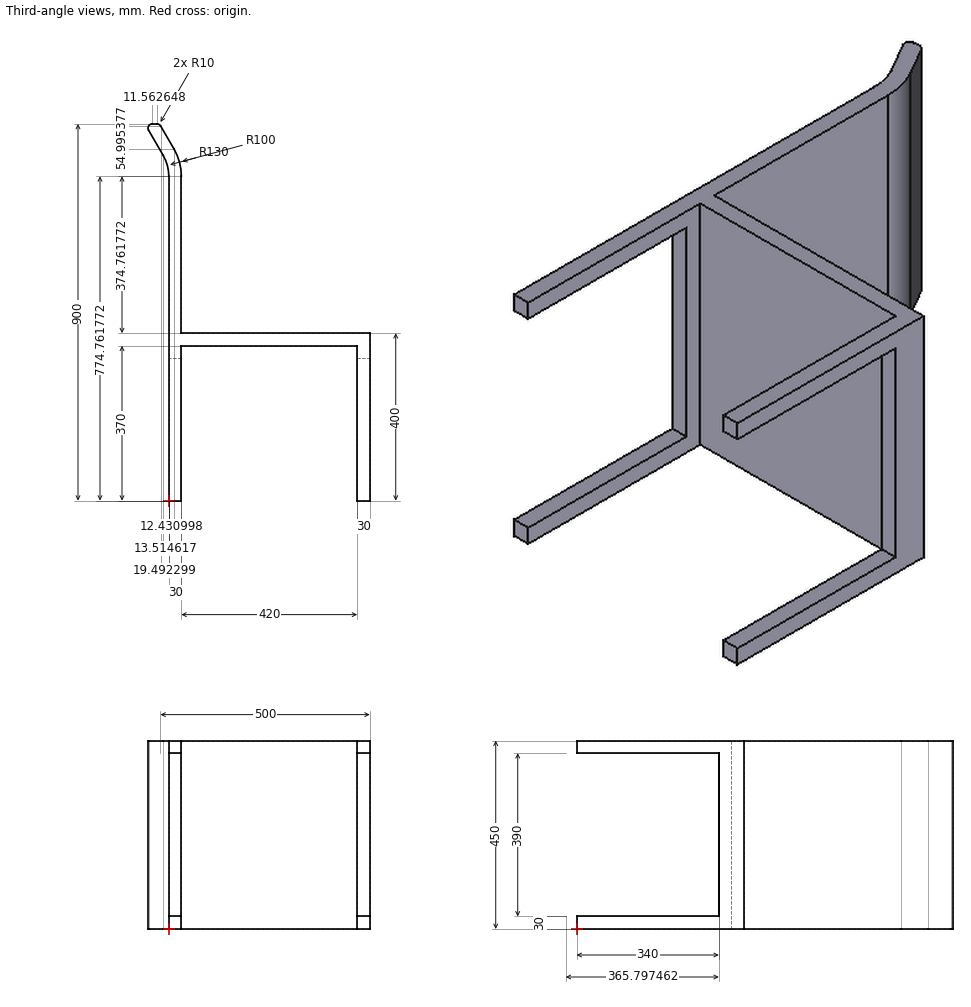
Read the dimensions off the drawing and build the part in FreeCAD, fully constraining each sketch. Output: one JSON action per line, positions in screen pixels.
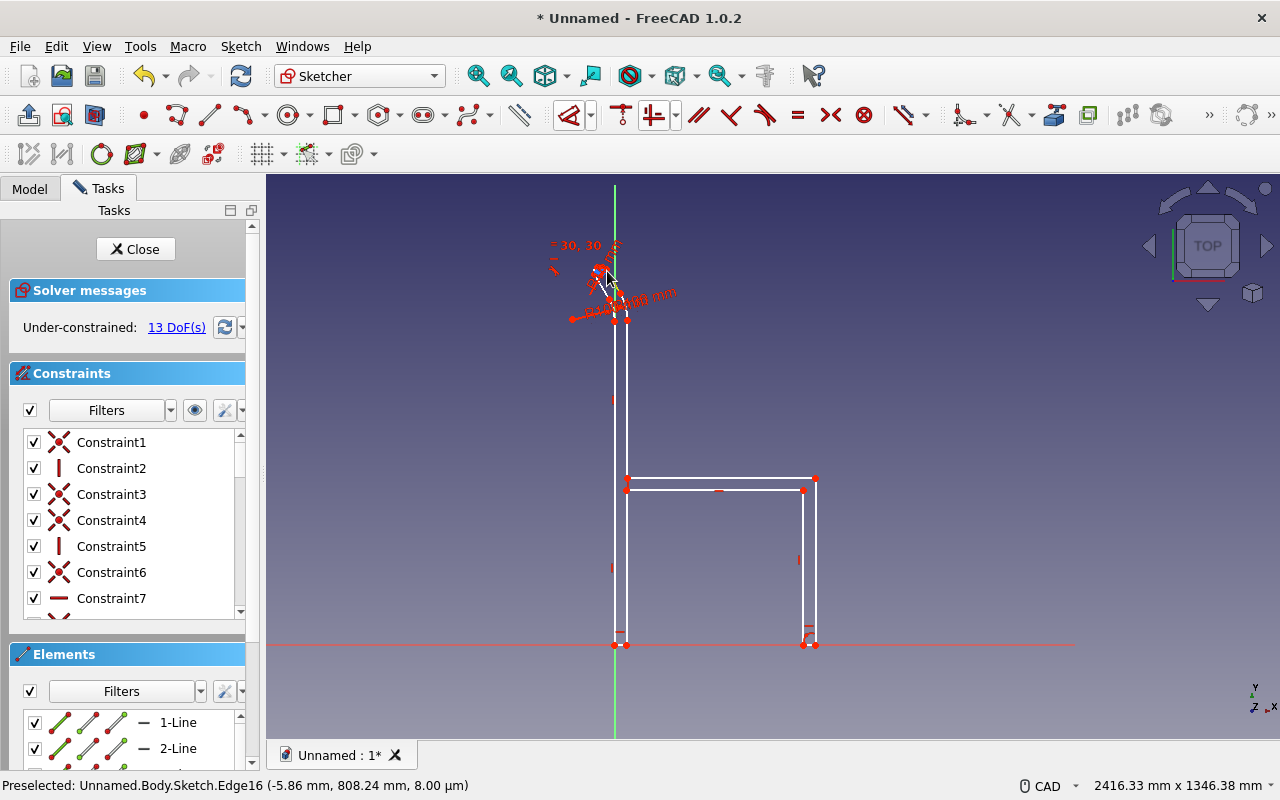
{"action": "scroll", "coordinate": [618, 645], "scroll_direction": "up", "scroll_amount": 7}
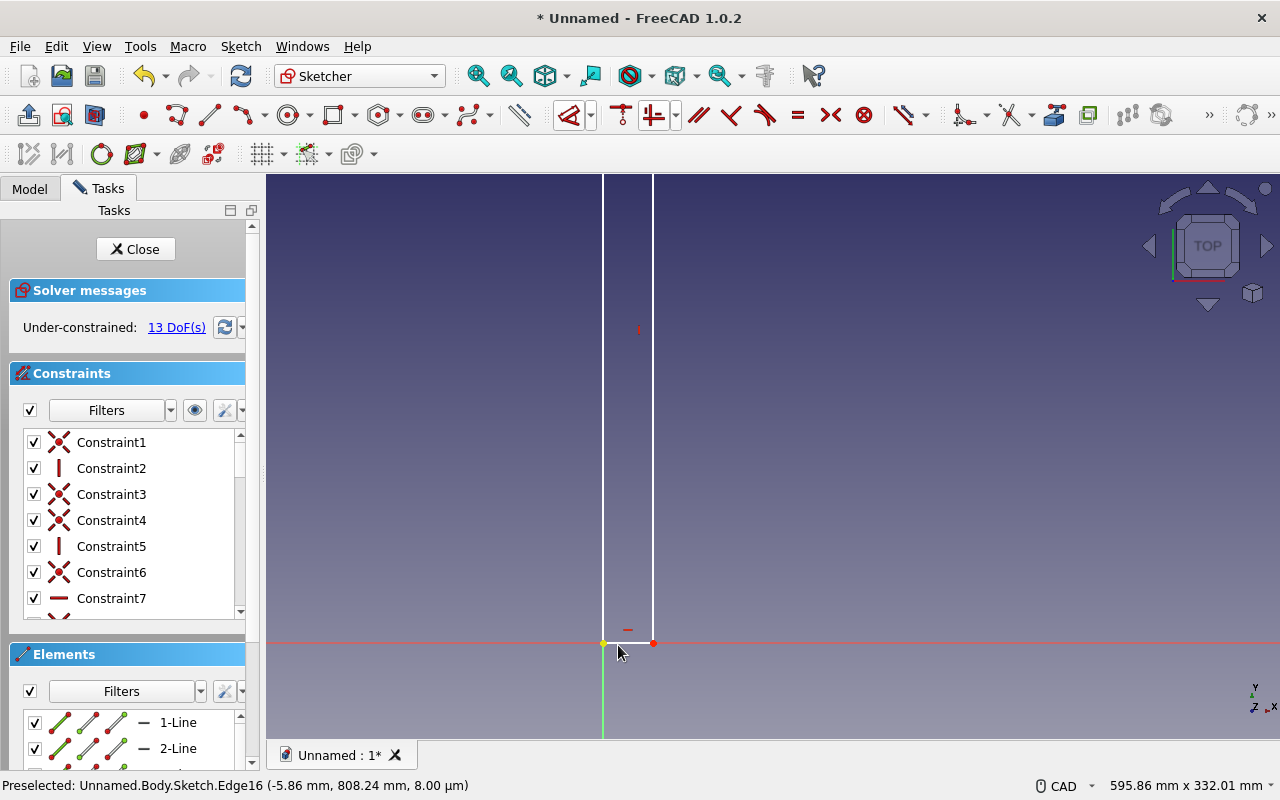
{"action": "left_click", "coordinate": [618, 643]}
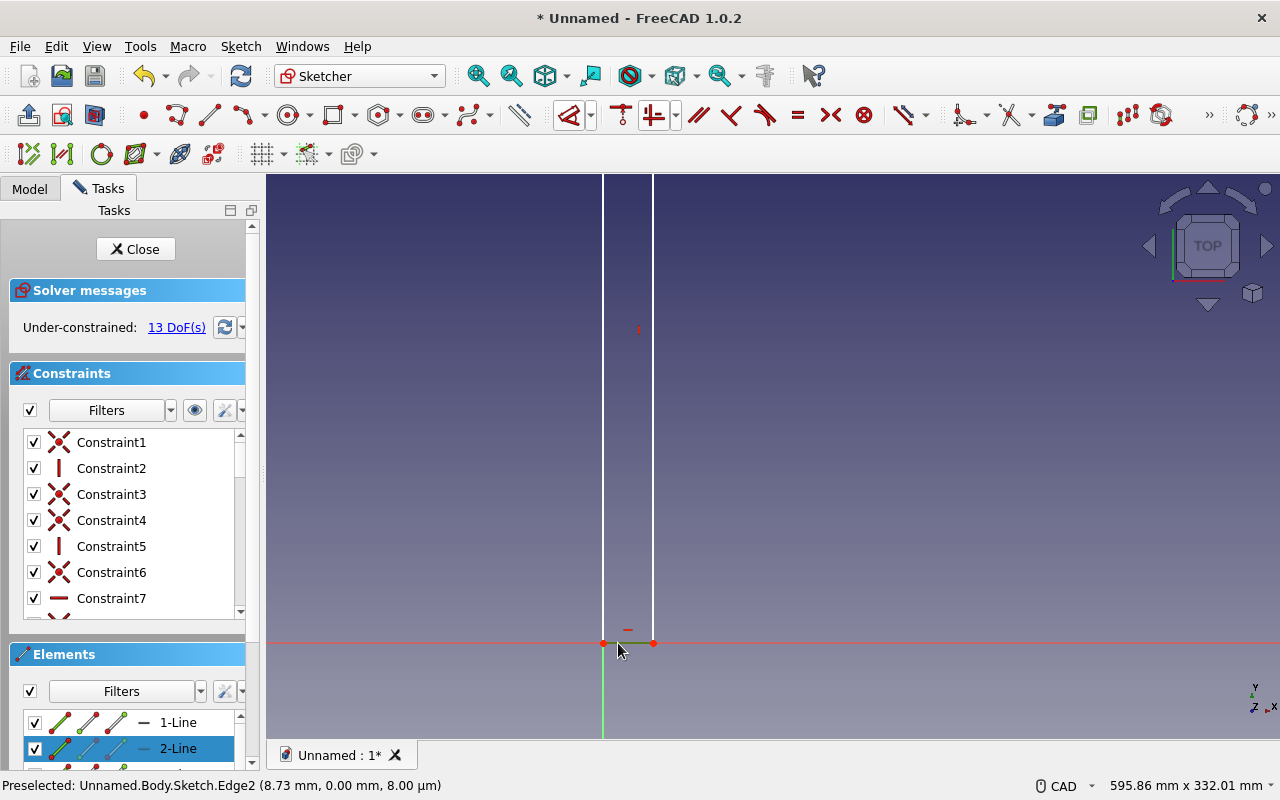
{"action": "key", "text": "l"}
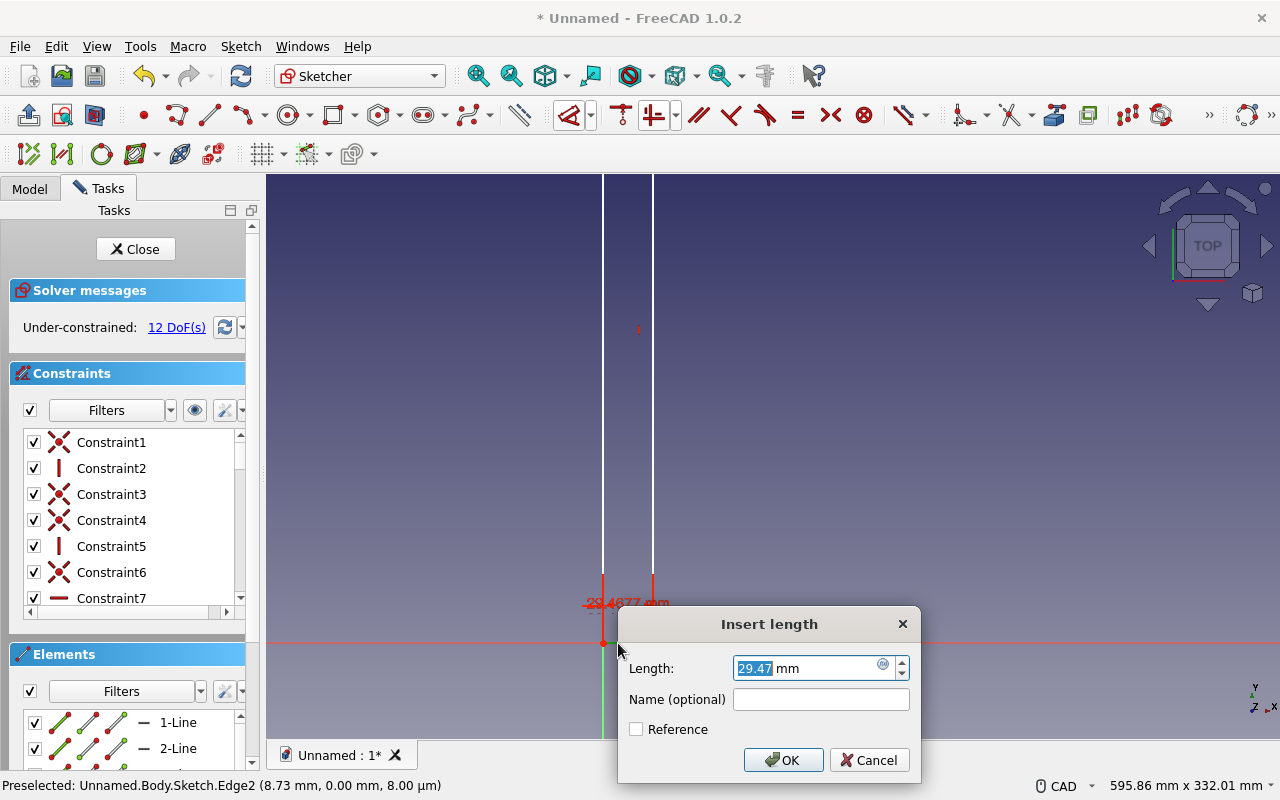
{"action": "type", "text": "30"}
{"action": "key", "text": "Return"}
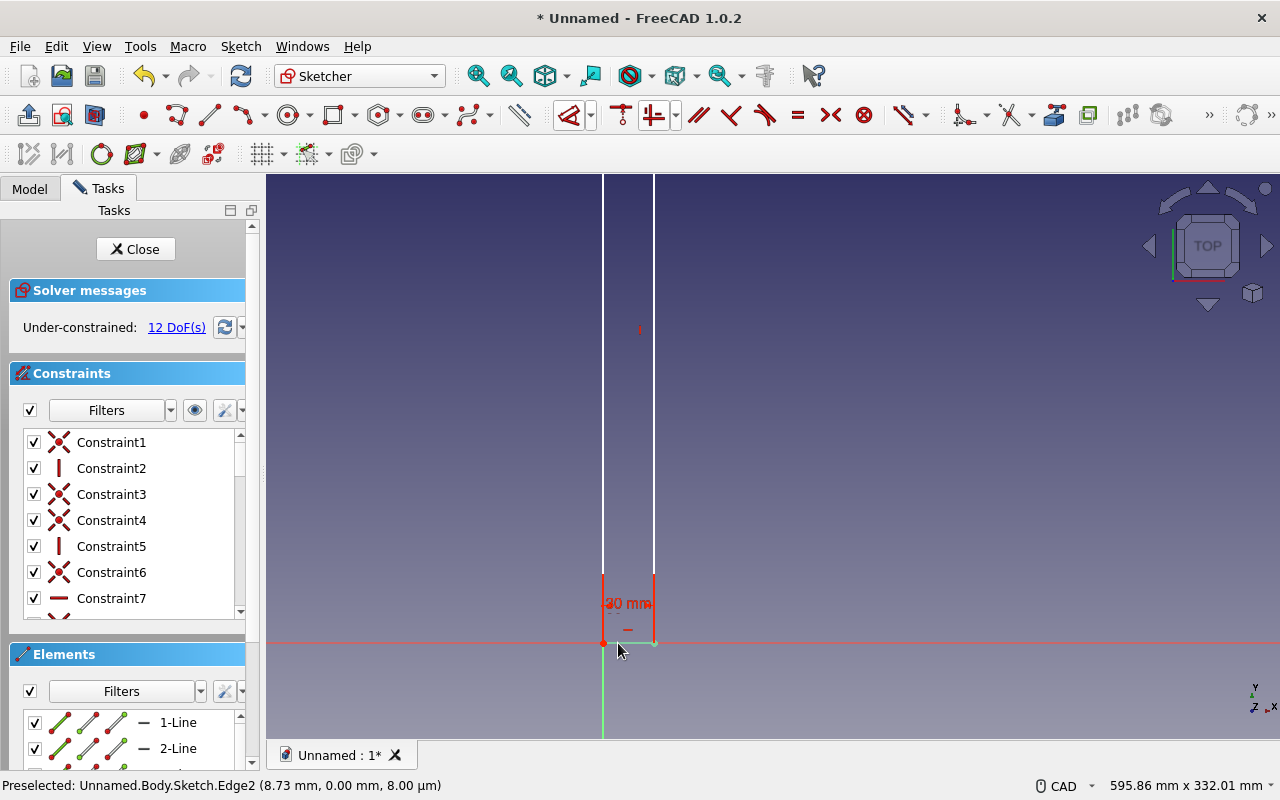
{"action": "scroll", "coordinate": [617, 646], "scroll_direction": "down", "scroll_amount": 7}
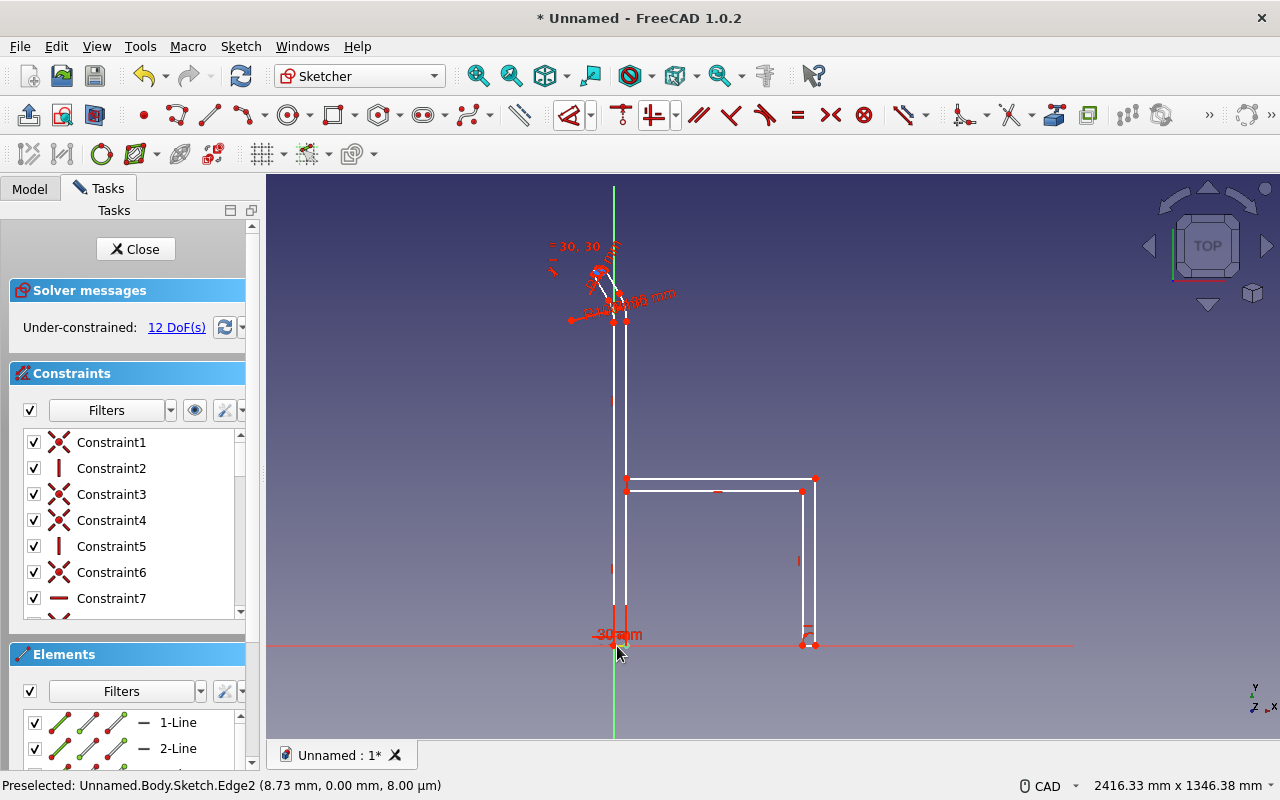
{"action": "scroll", "coordinate": [806, 646], "scroll_direction": "up", "scroll_amount": 7}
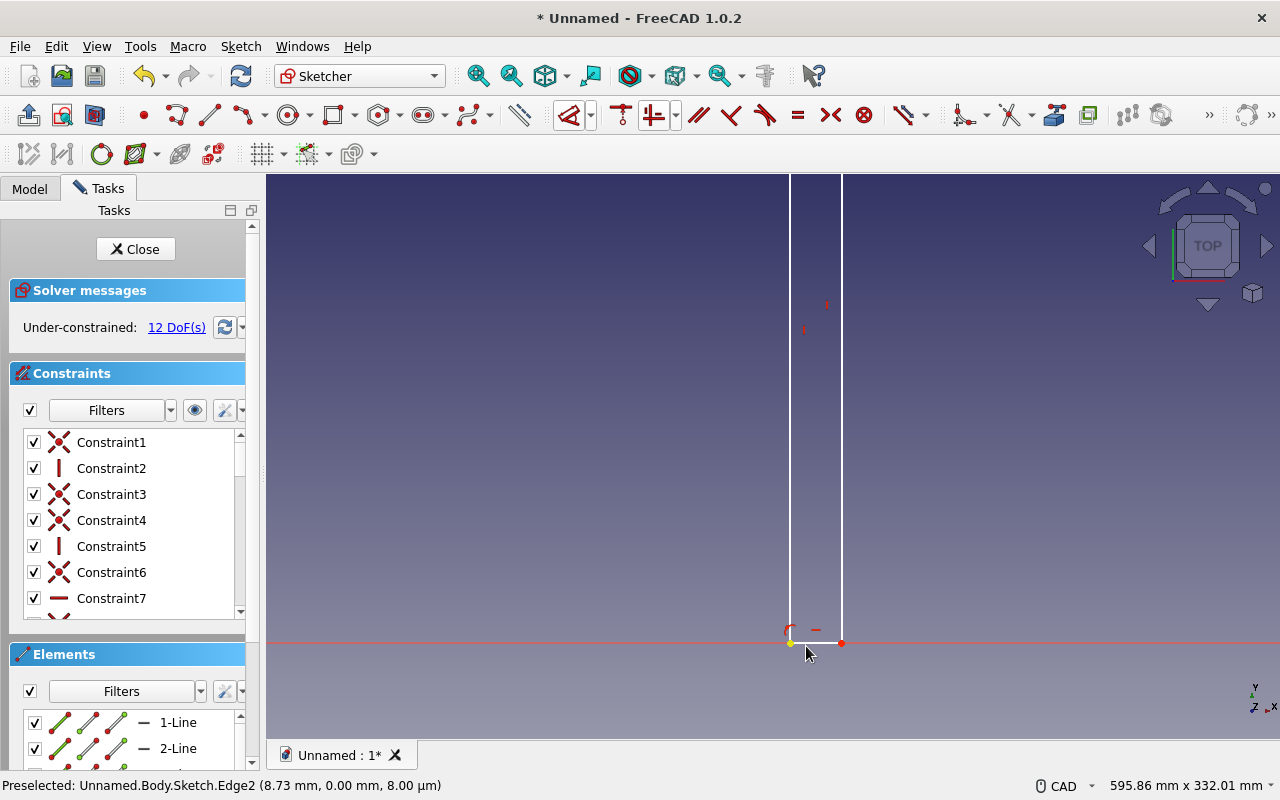
{"action": "left_click", "coordinate": [806, 643]}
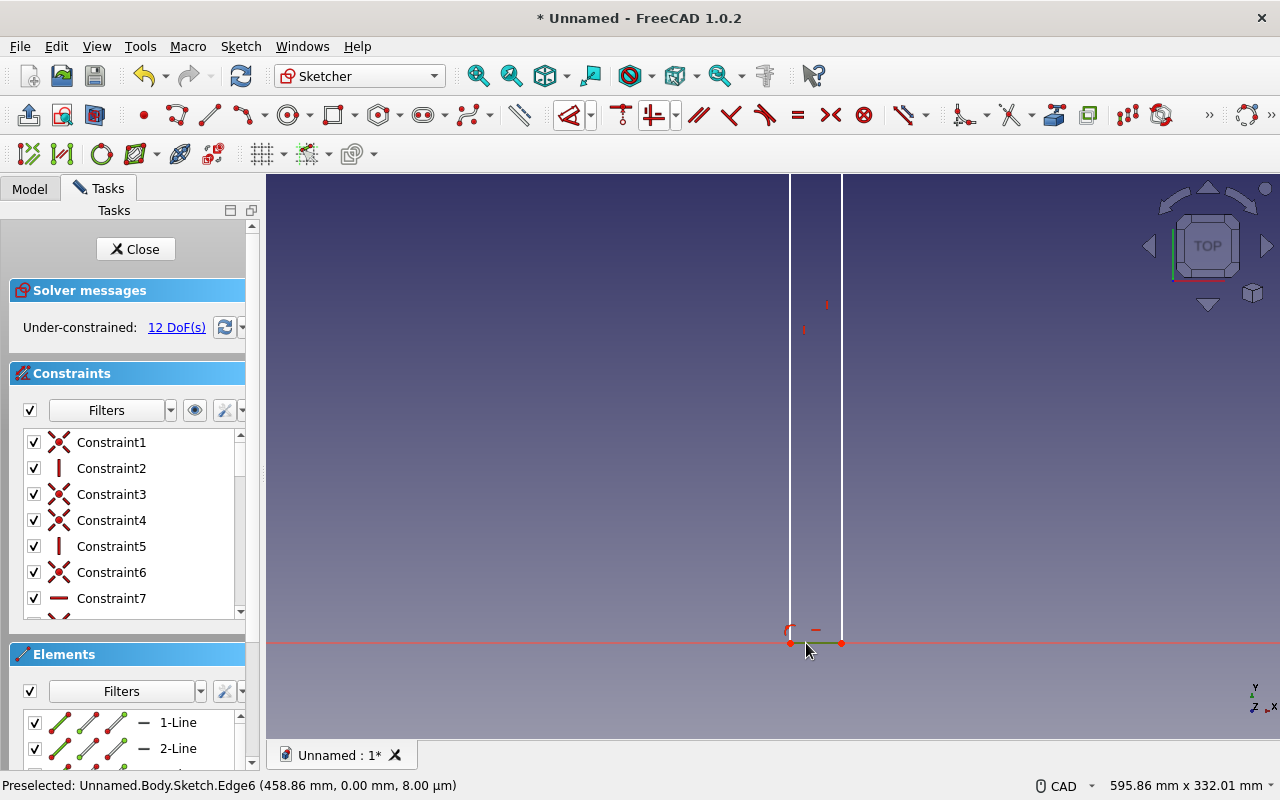
{"action": "key", "text": "l"}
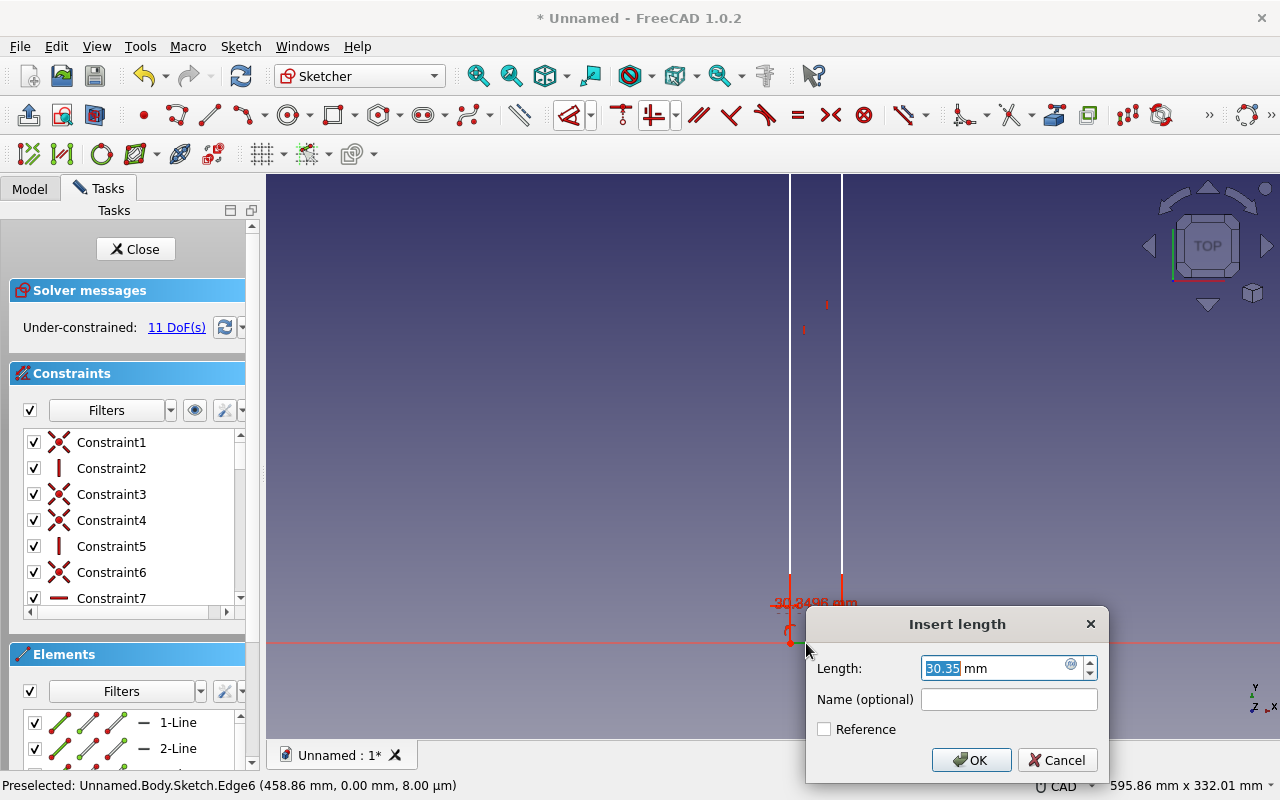
{"action": "type", "text": "30"}
{"action": "key", "text": "Return"}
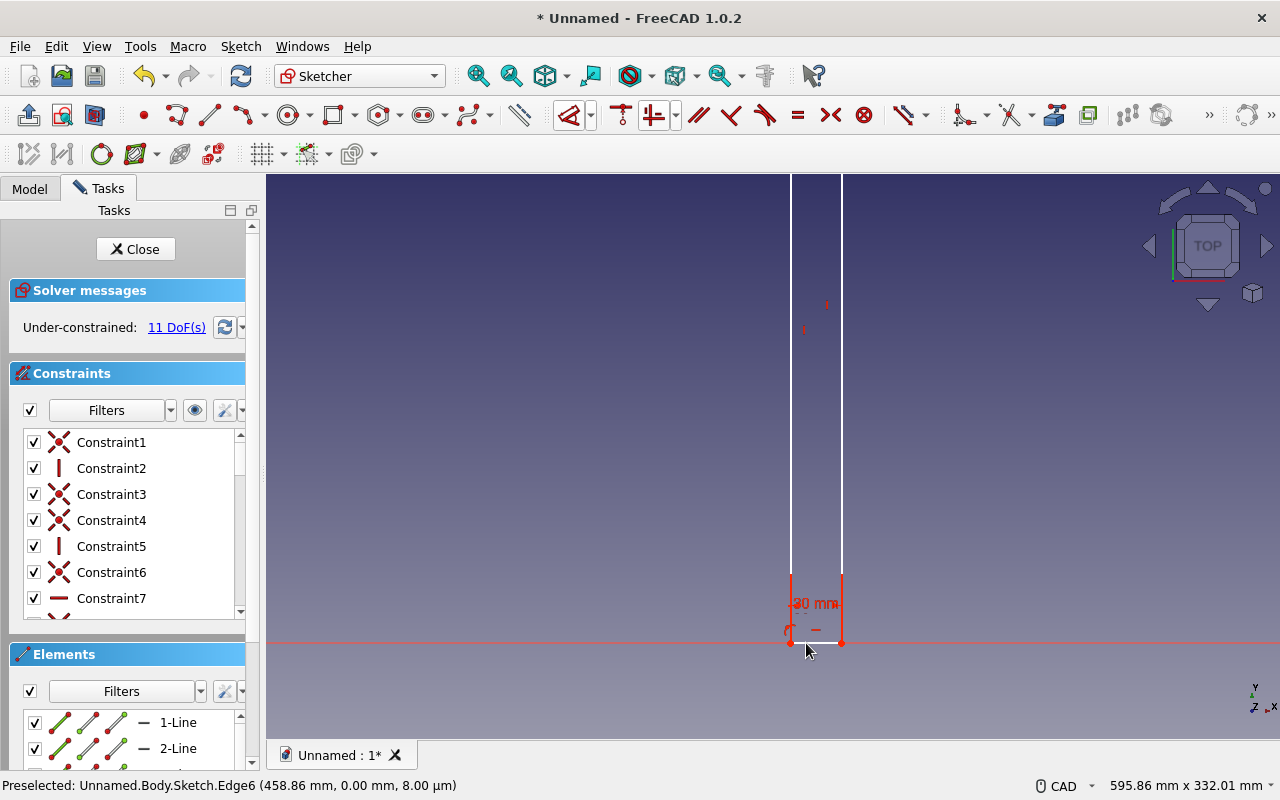
{"action": "scroll", "coordinate": [807, 646], "scroll_direction": "down", "scroll_amount": 7}